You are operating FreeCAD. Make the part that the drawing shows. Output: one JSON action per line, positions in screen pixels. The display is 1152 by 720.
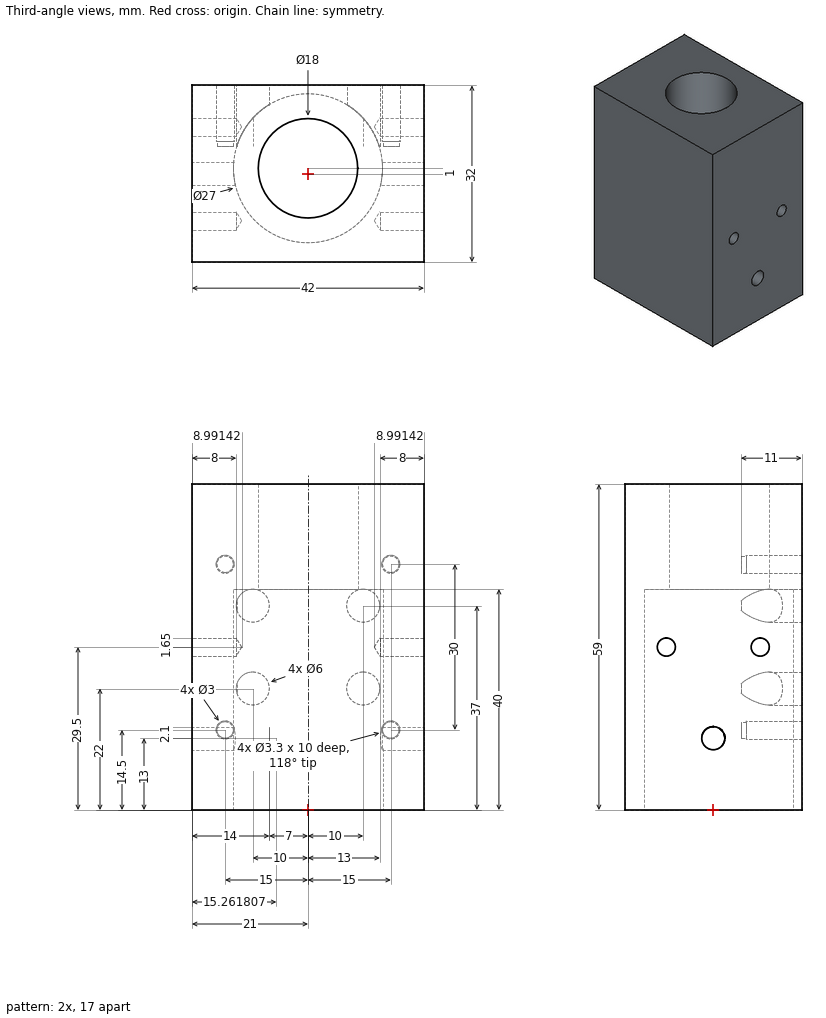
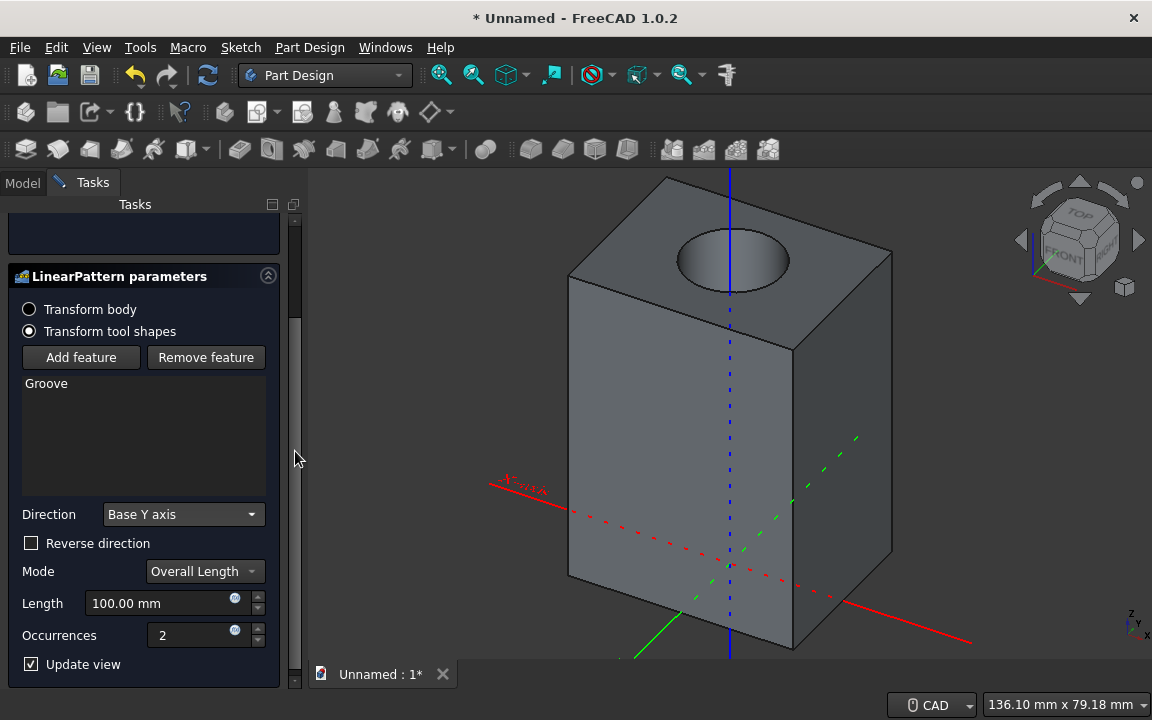
{"action": "left_click", "coordinate": [206, 572]}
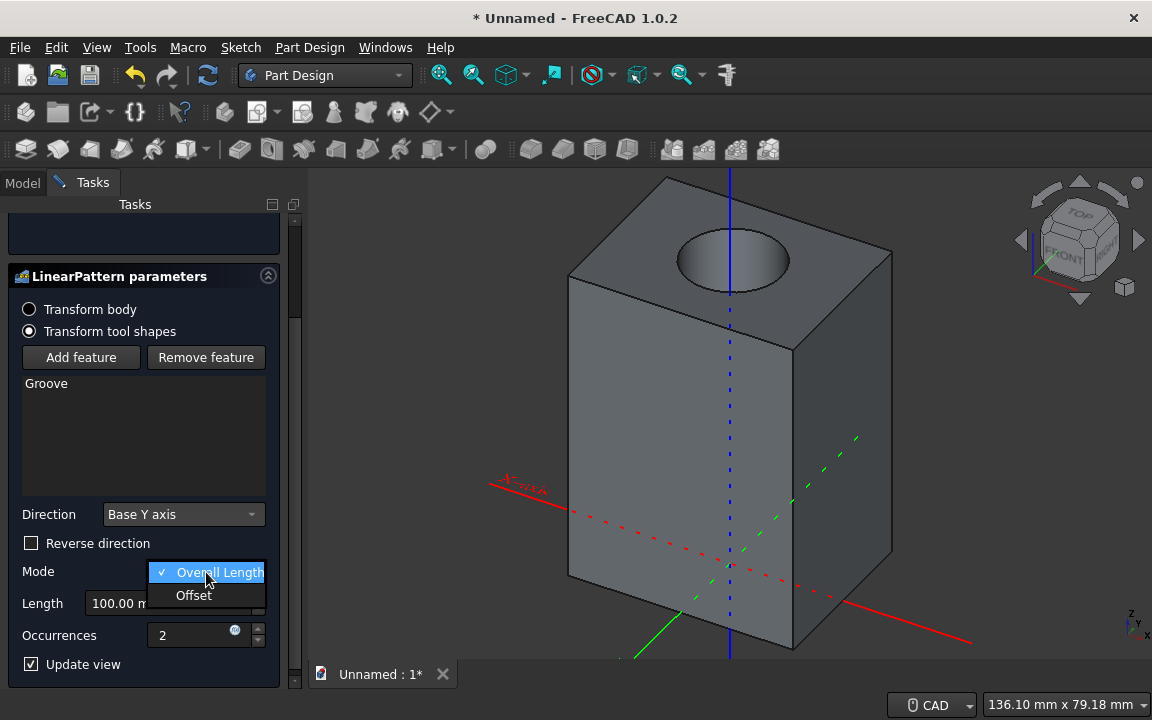
{"action": "left_click", "coordinate": [206, 596]}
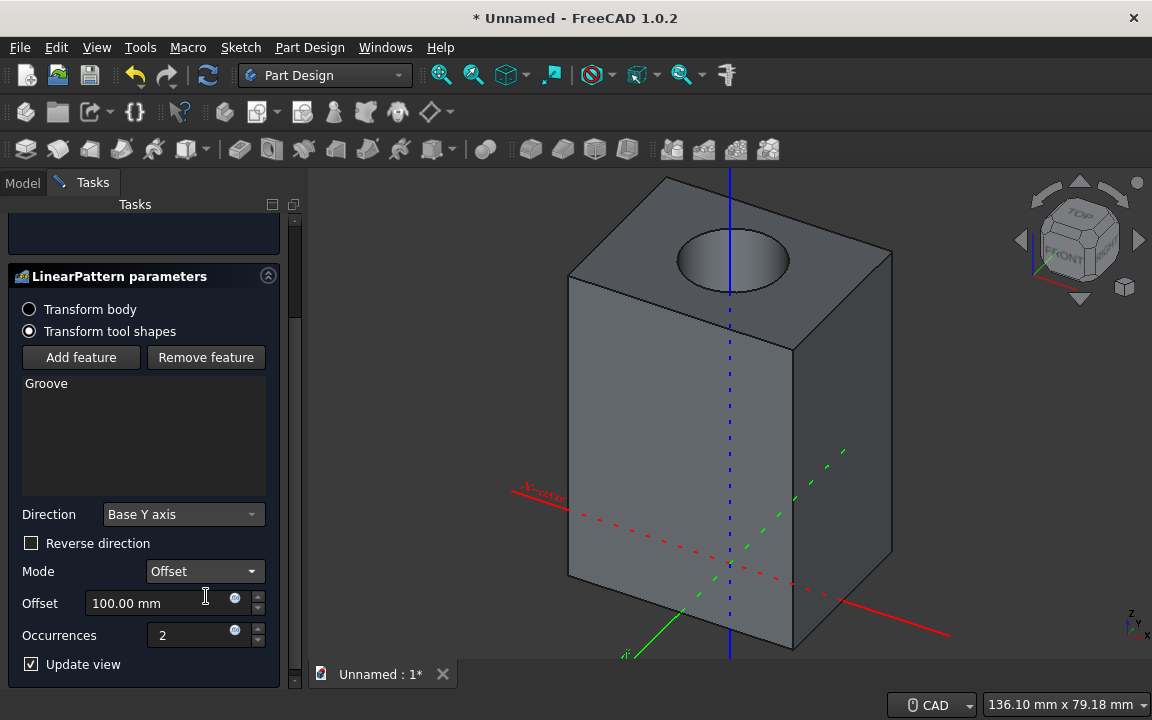
{"action": "triple_click", "coordinate": [168, 603]}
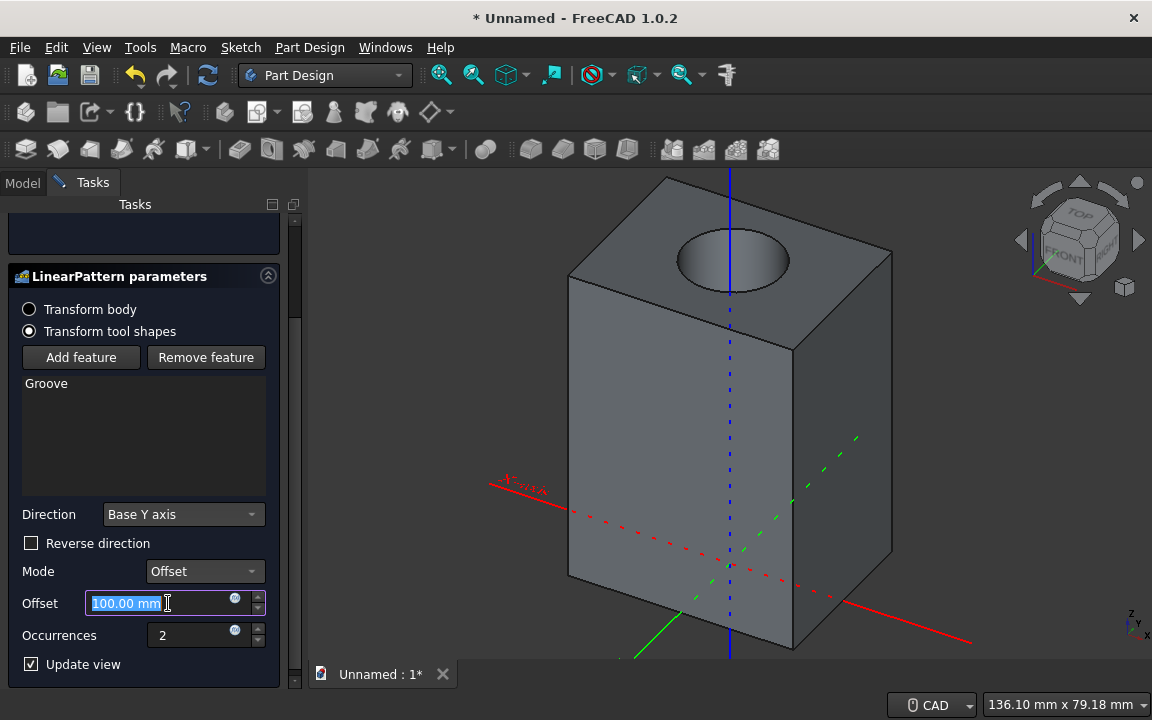
{"action": "type", "text": "17"}
{"action": "key", "text": "Tab"}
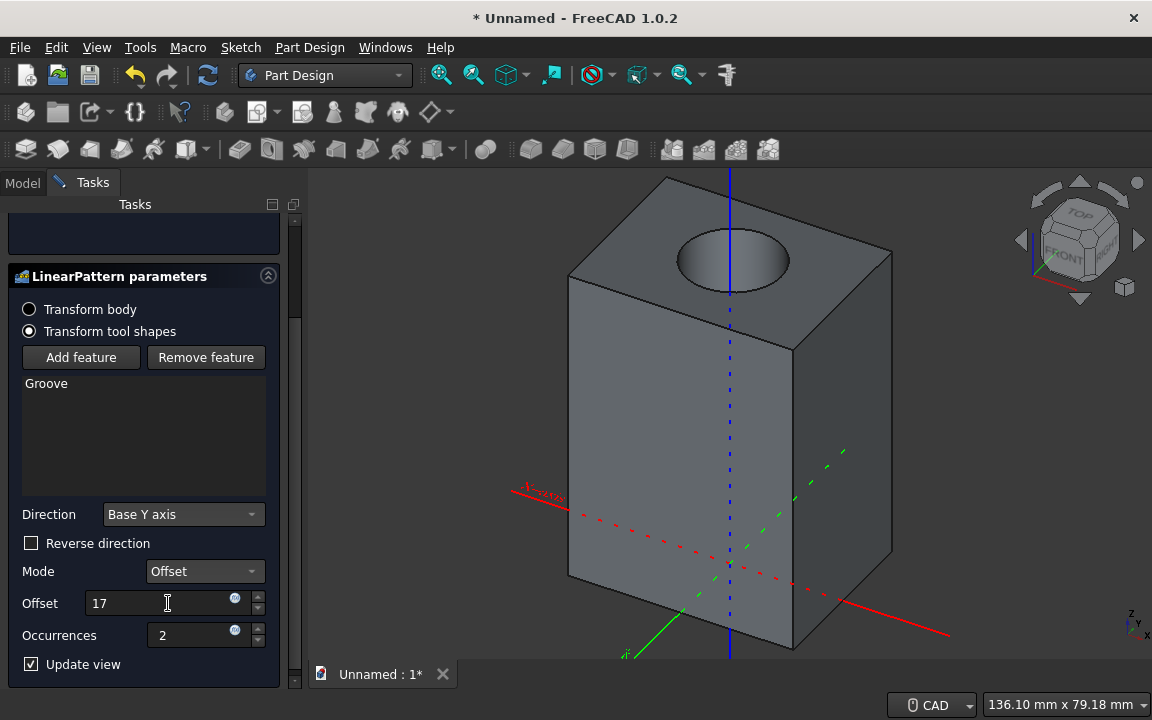
{"action": "triple_click", "coordinate": [198, 635]}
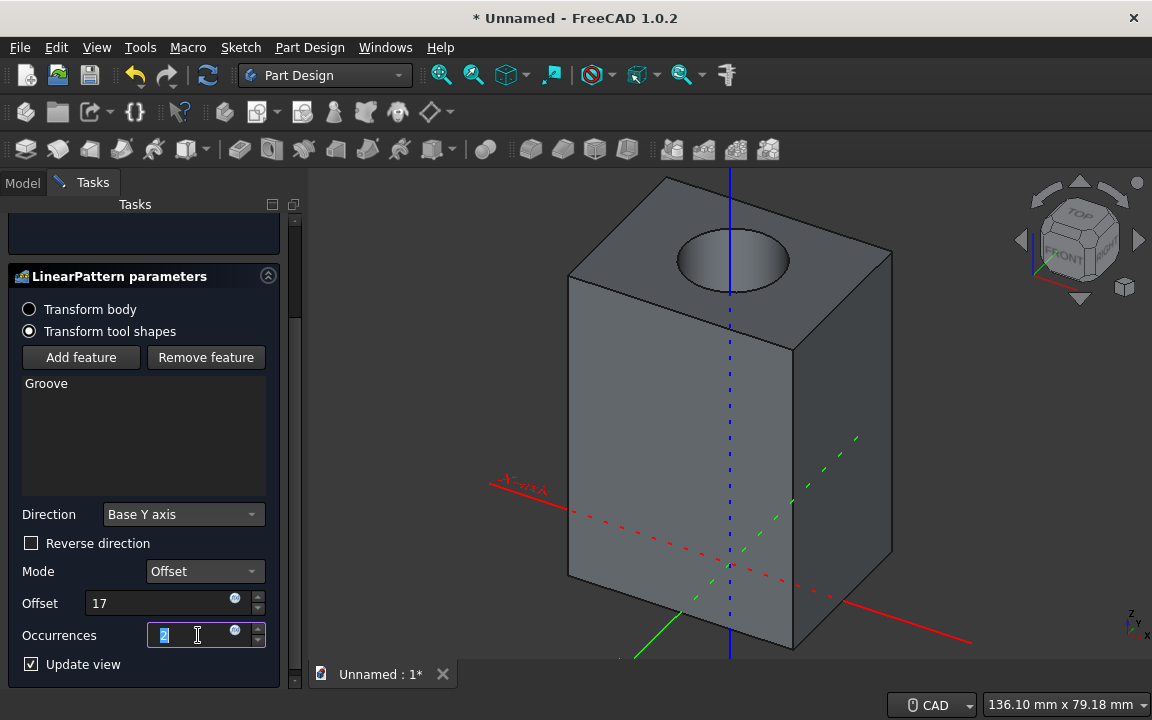
{"action": "type", "text": "2"}
{"action": "key", "text": "Tab"}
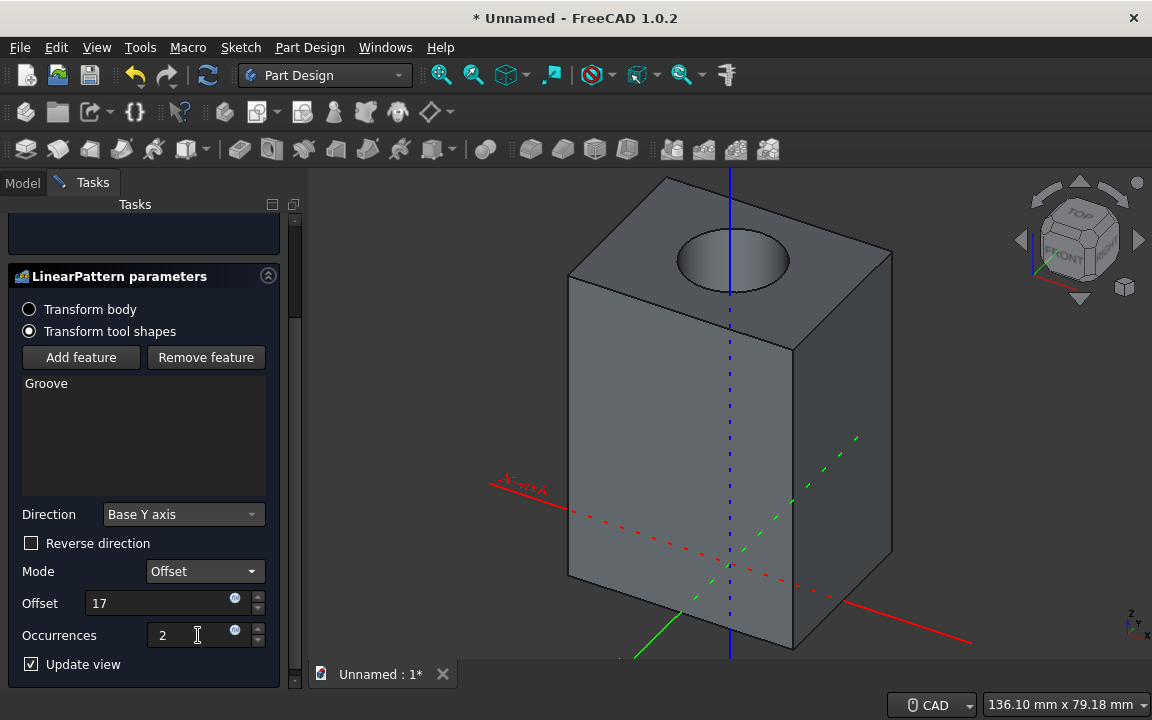
{"action": "left_click", "coordinate": [30, 543]}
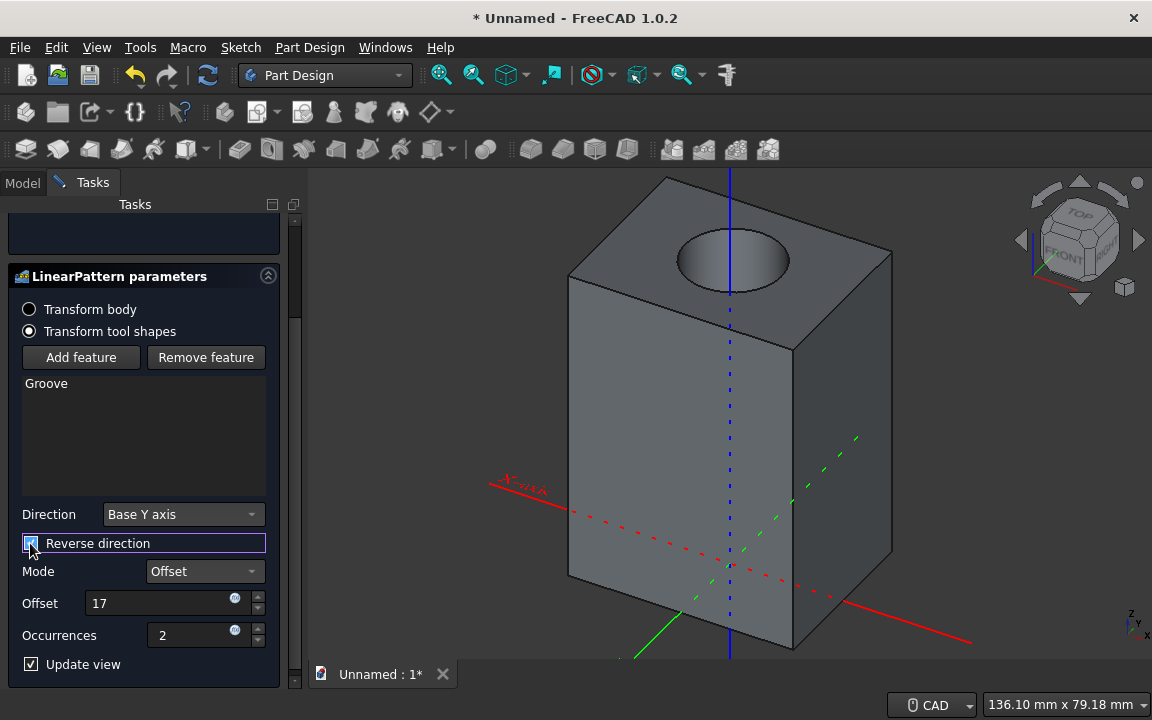
{"action": "scroll", "coordinate": [295, 451], "scroll_direction": "up", "scroll_amount": 3}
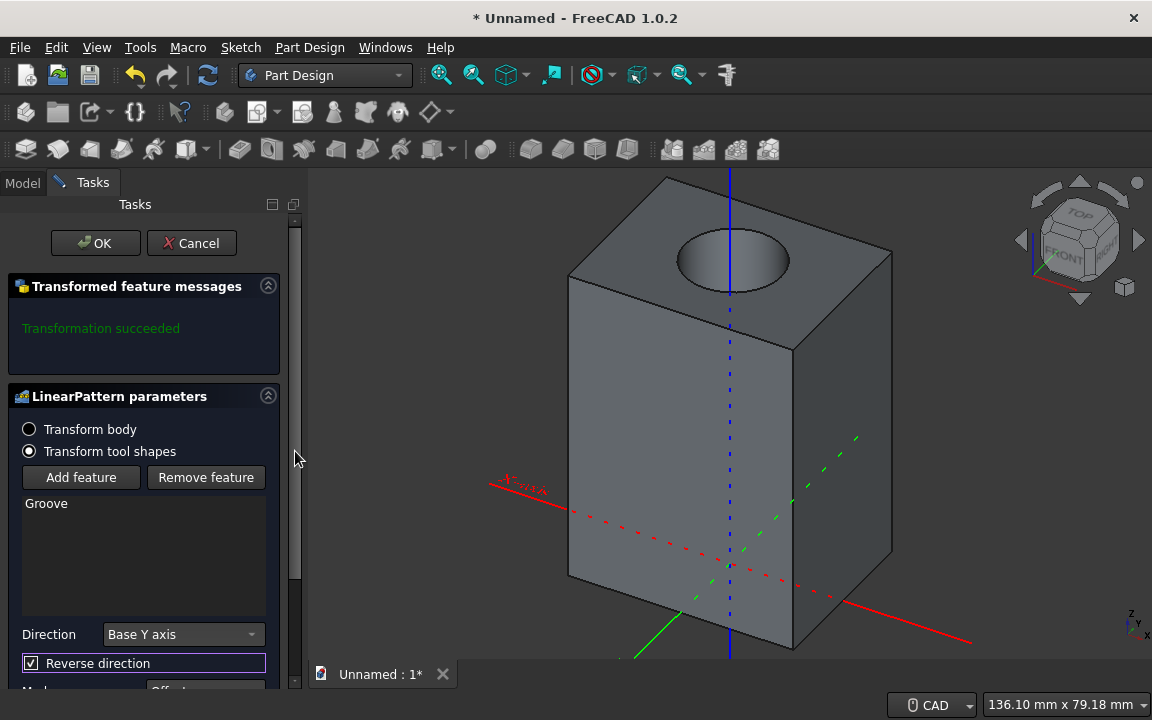
{"action": "left_click", "coordinate": [96, 243]}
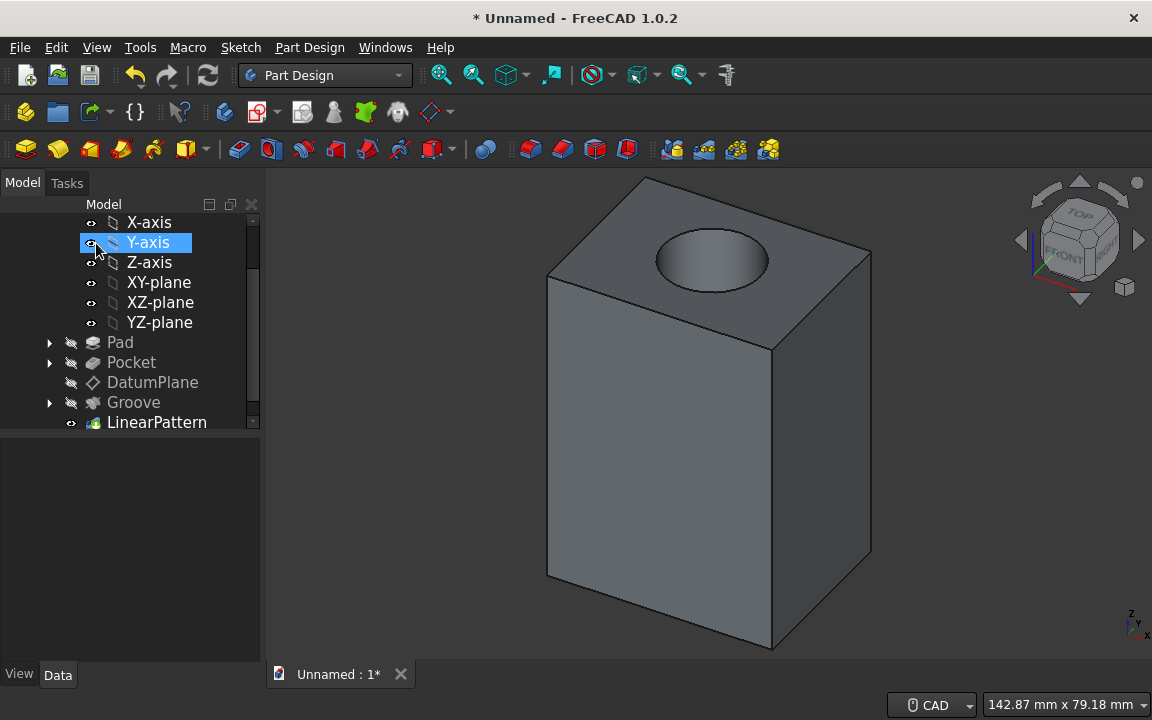
{"action": "left_click", "coordinate": [258, 112]}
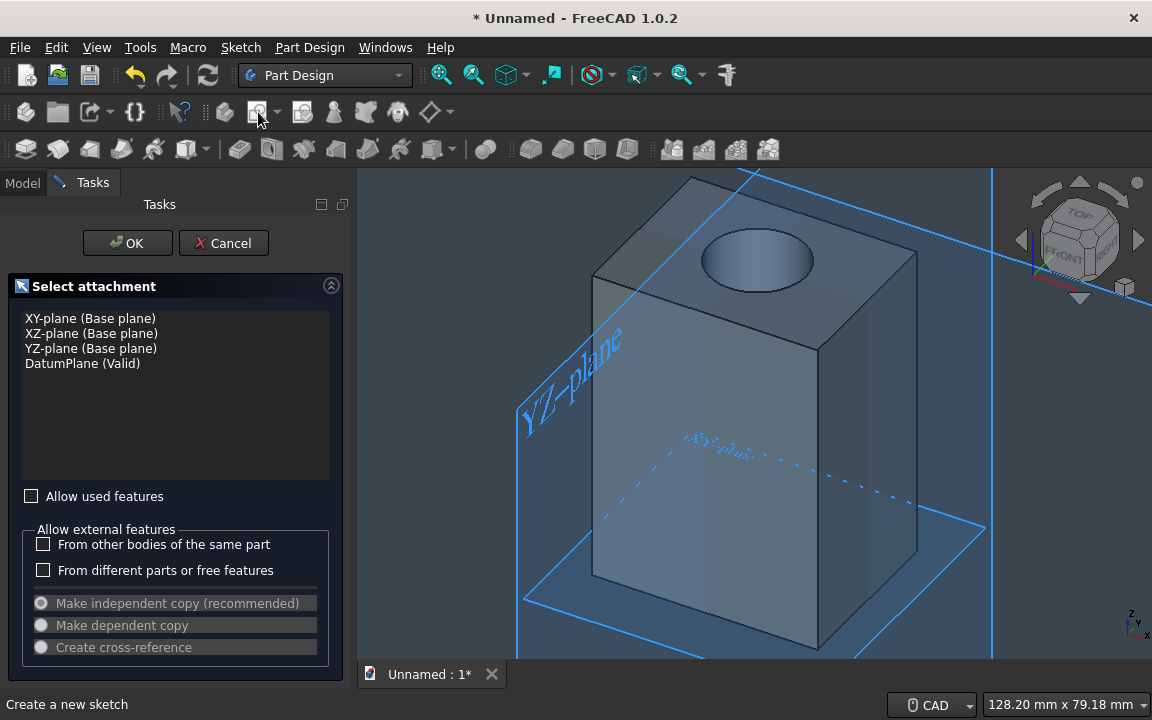
{"action": "left_click", "coordinate": [82, 334]}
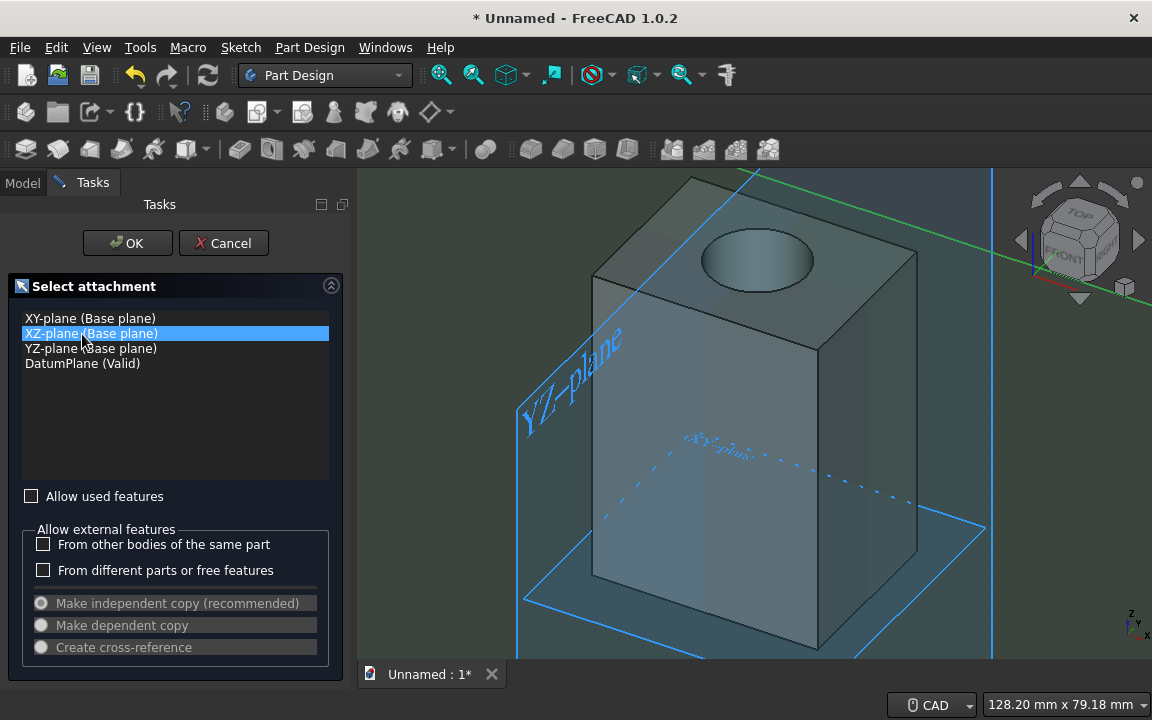
{"action": "left_click", "coordinate": [128, 243]}